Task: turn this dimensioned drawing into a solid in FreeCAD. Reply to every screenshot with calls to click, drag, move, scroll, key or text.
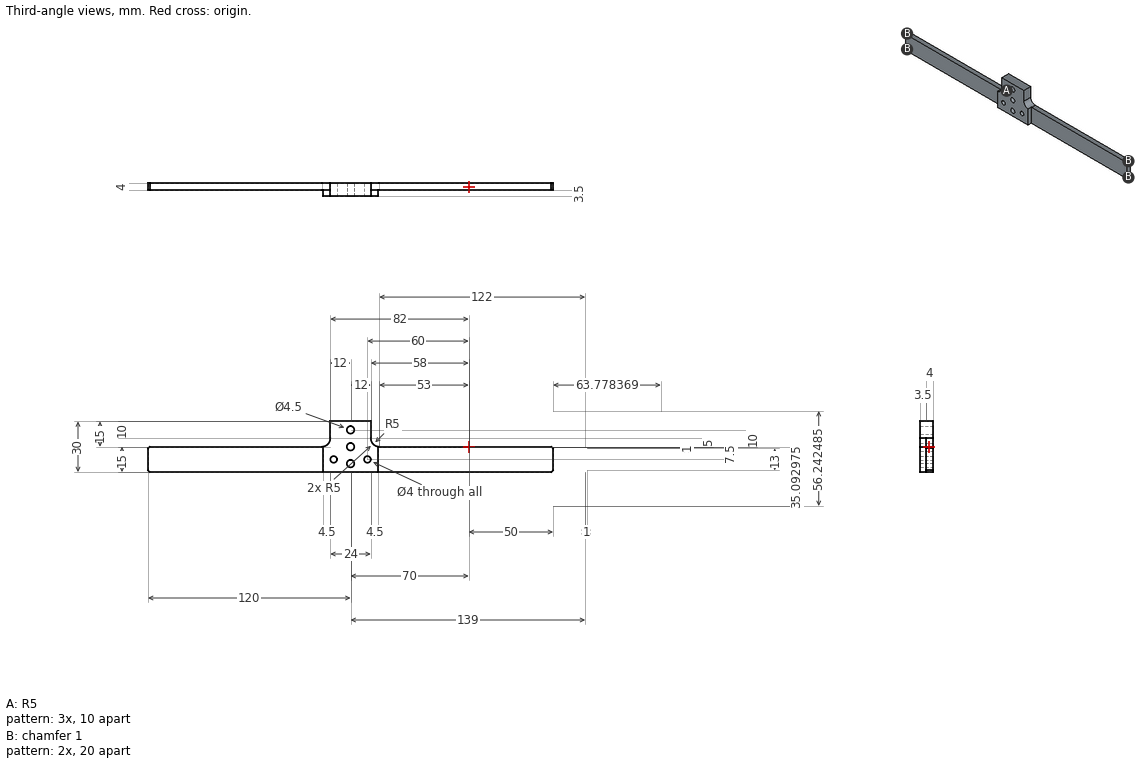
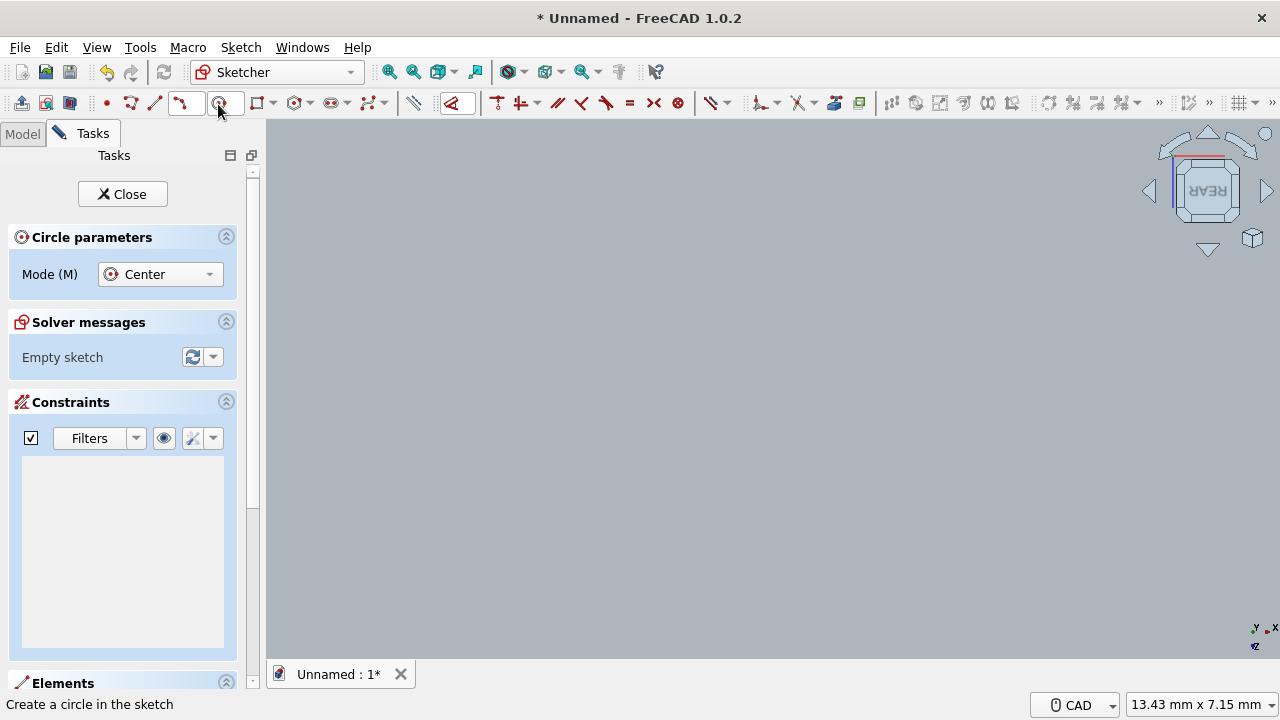
click(704, 389)
click(824, 269)
key(Escape)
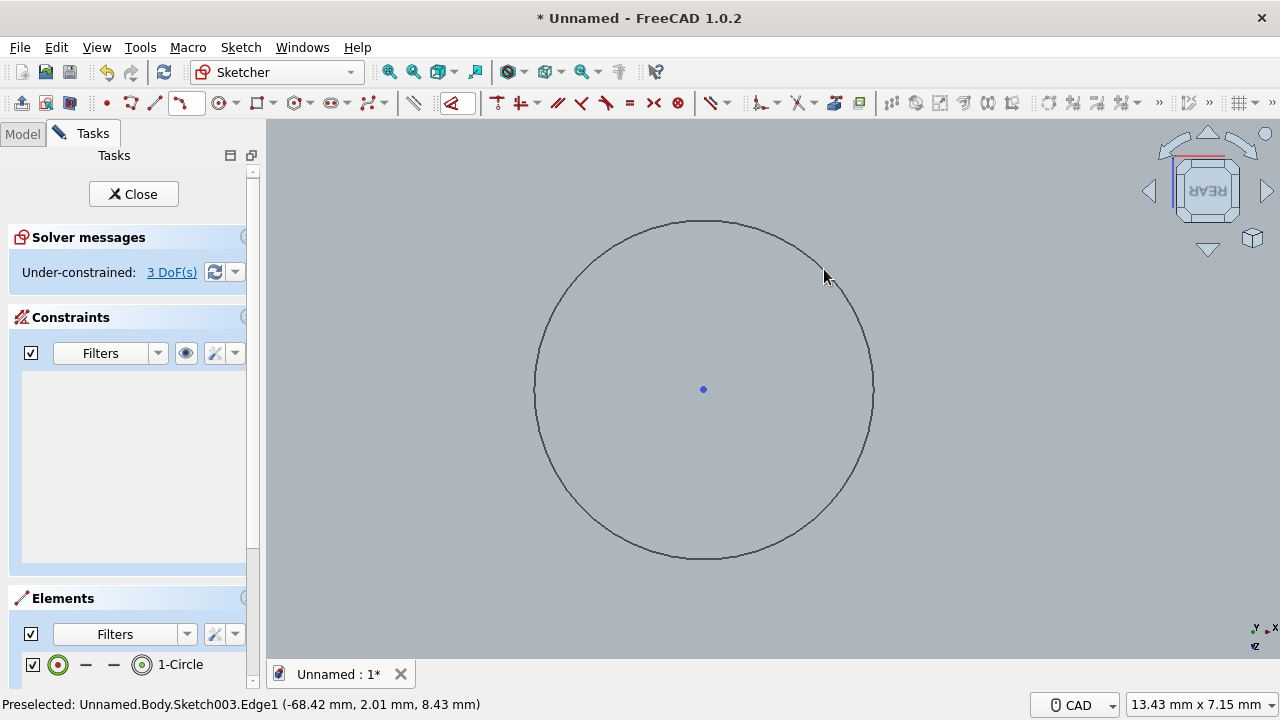
click(824, 270)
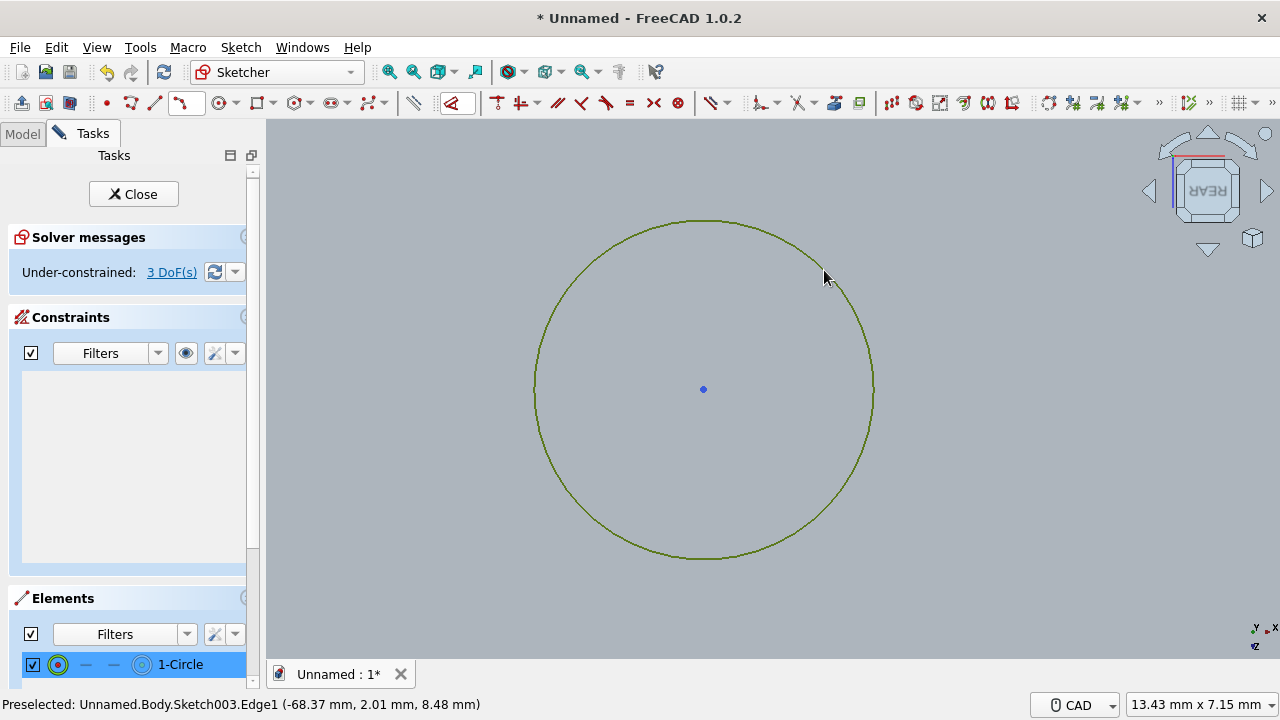
key(k)
key(o)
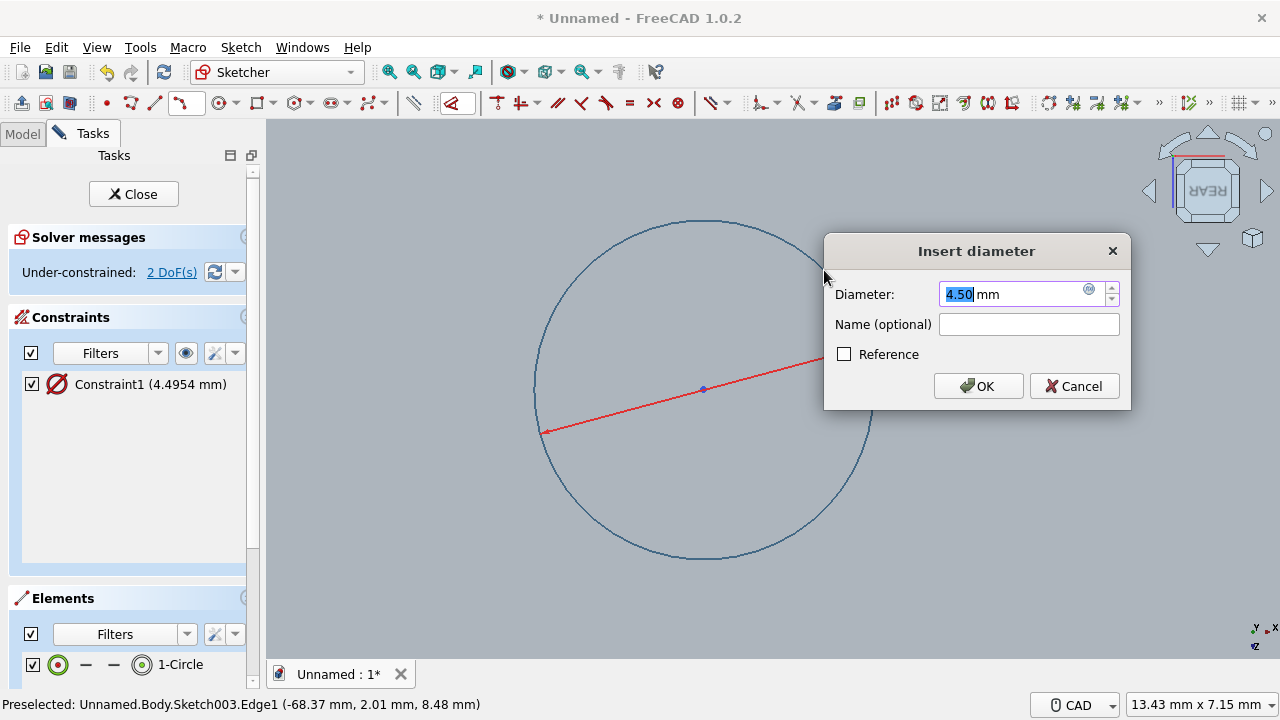
text(4.5)
key(Return)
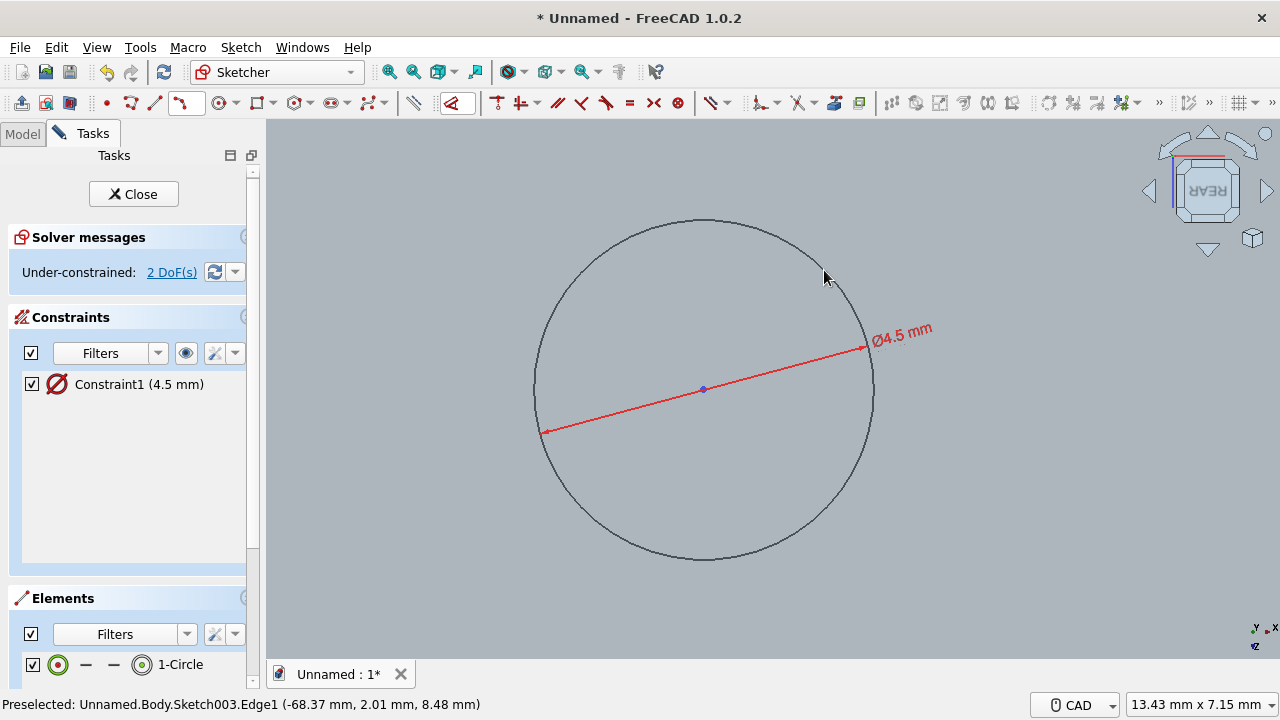
click(704, 390)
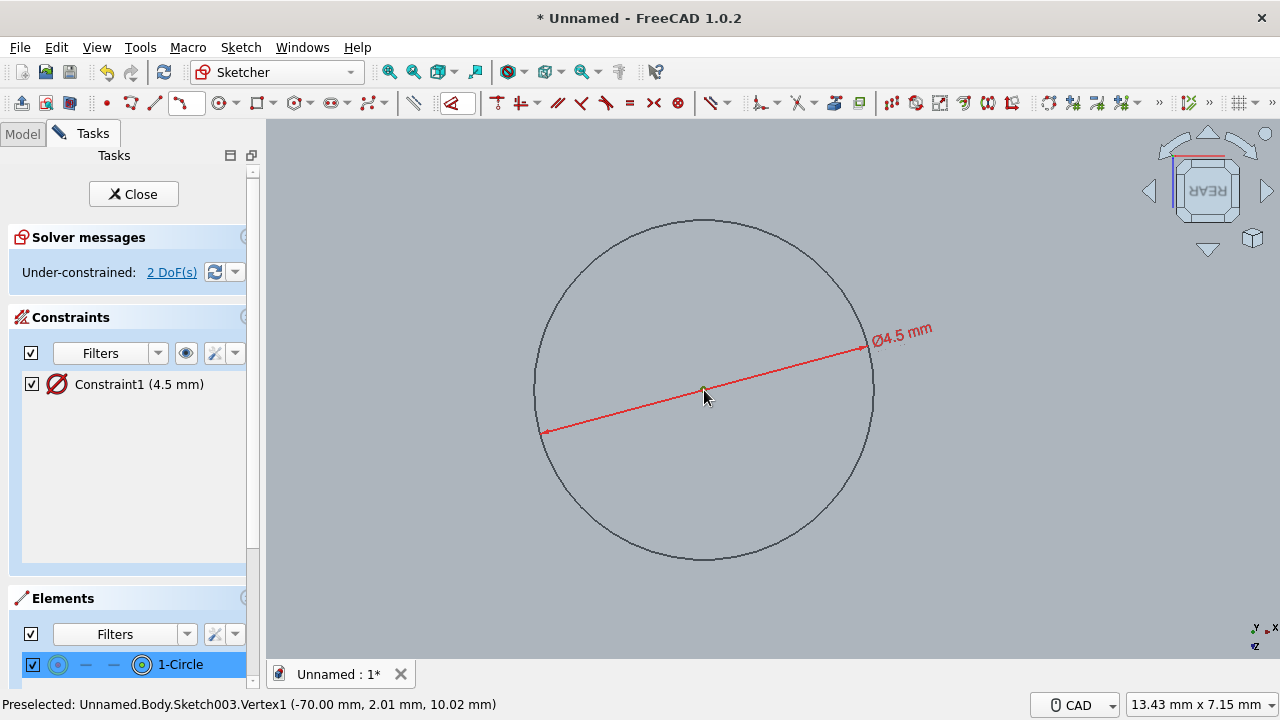
click(470, 104)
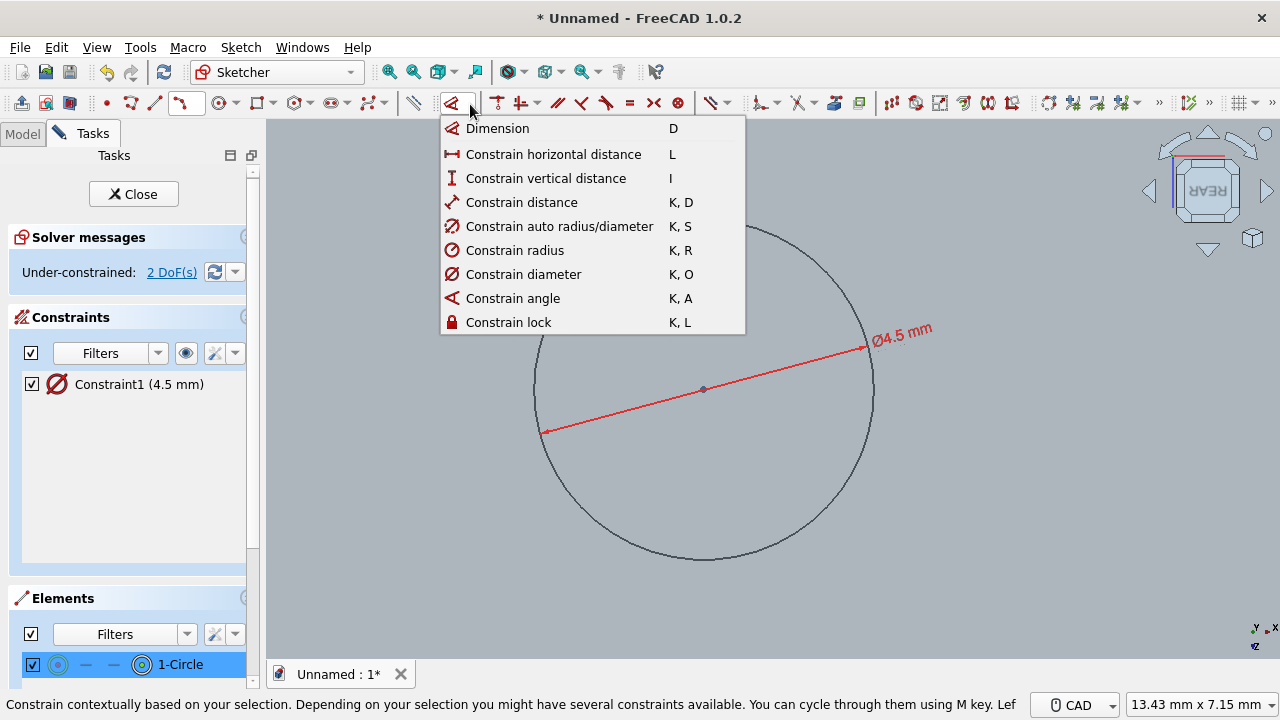
click(593, 154)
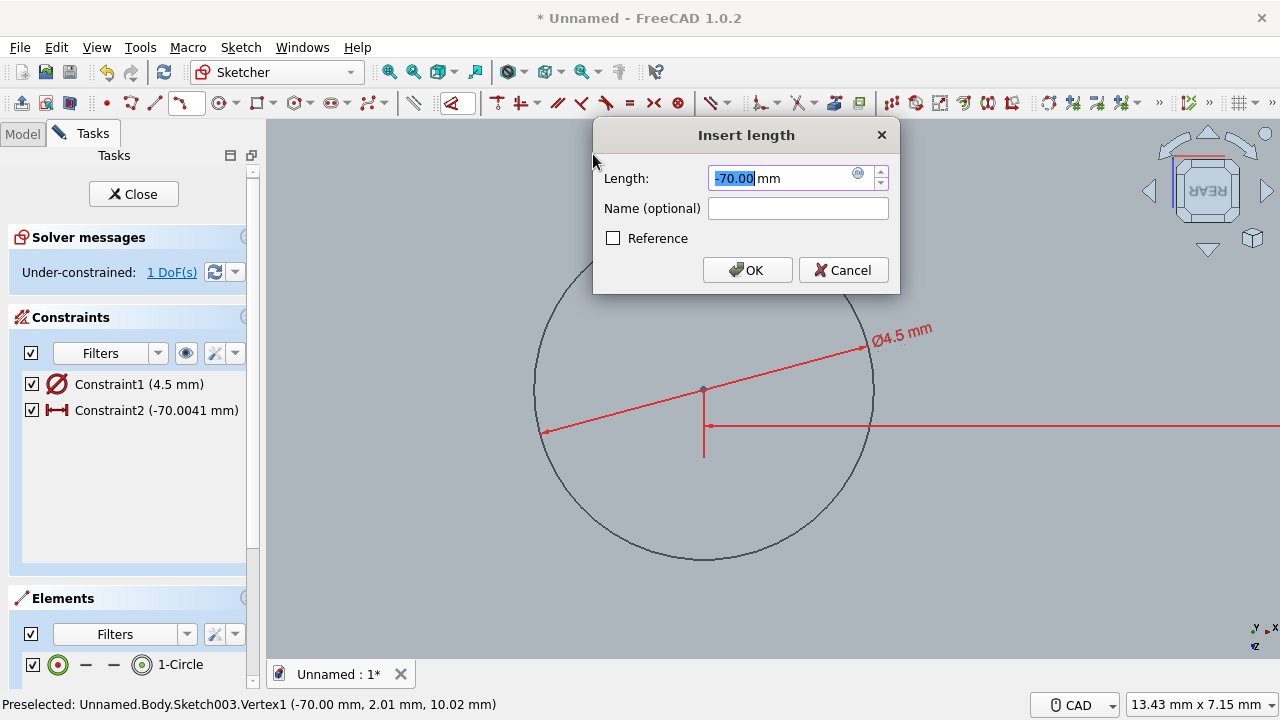
text(-70)
key(Return)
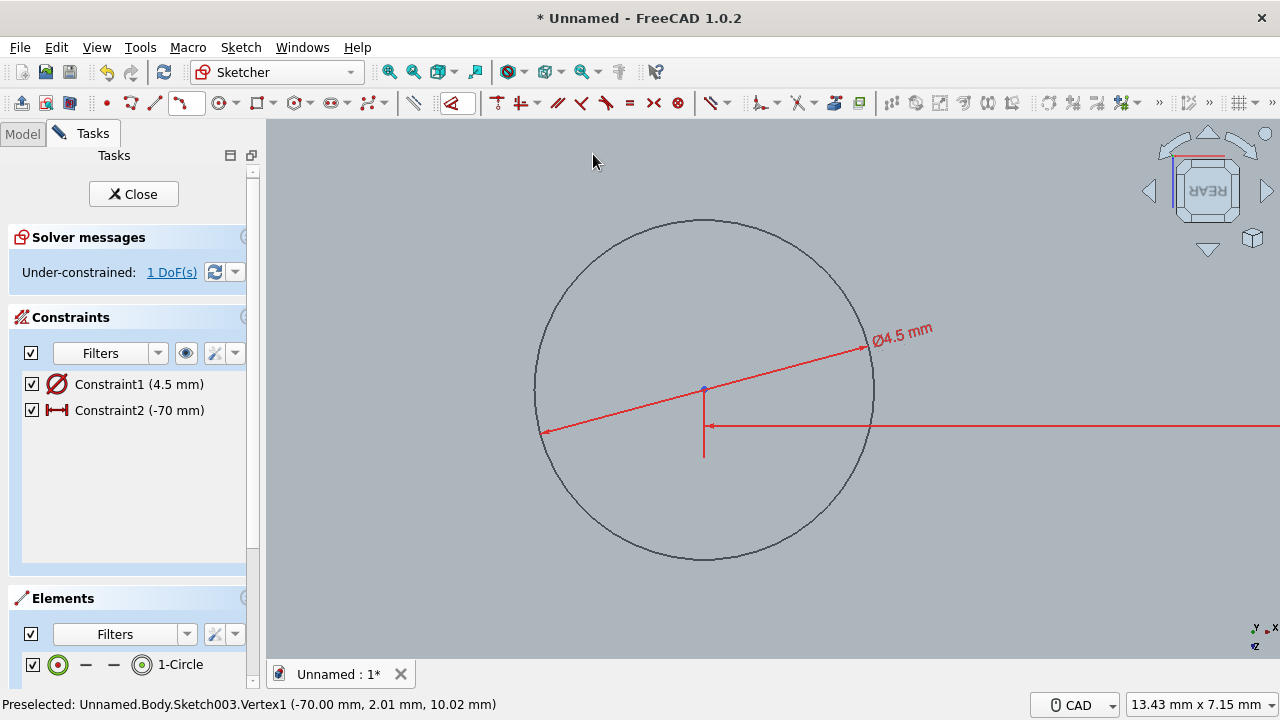
click(704, 390)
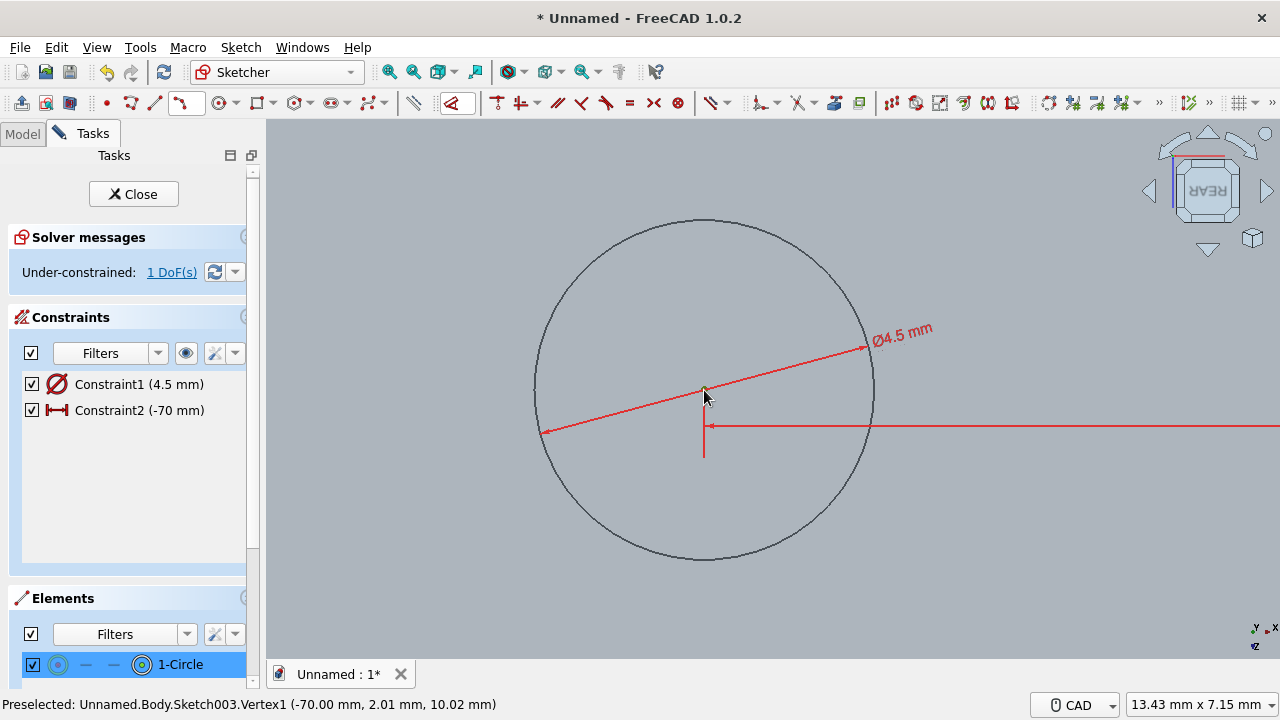
key(i)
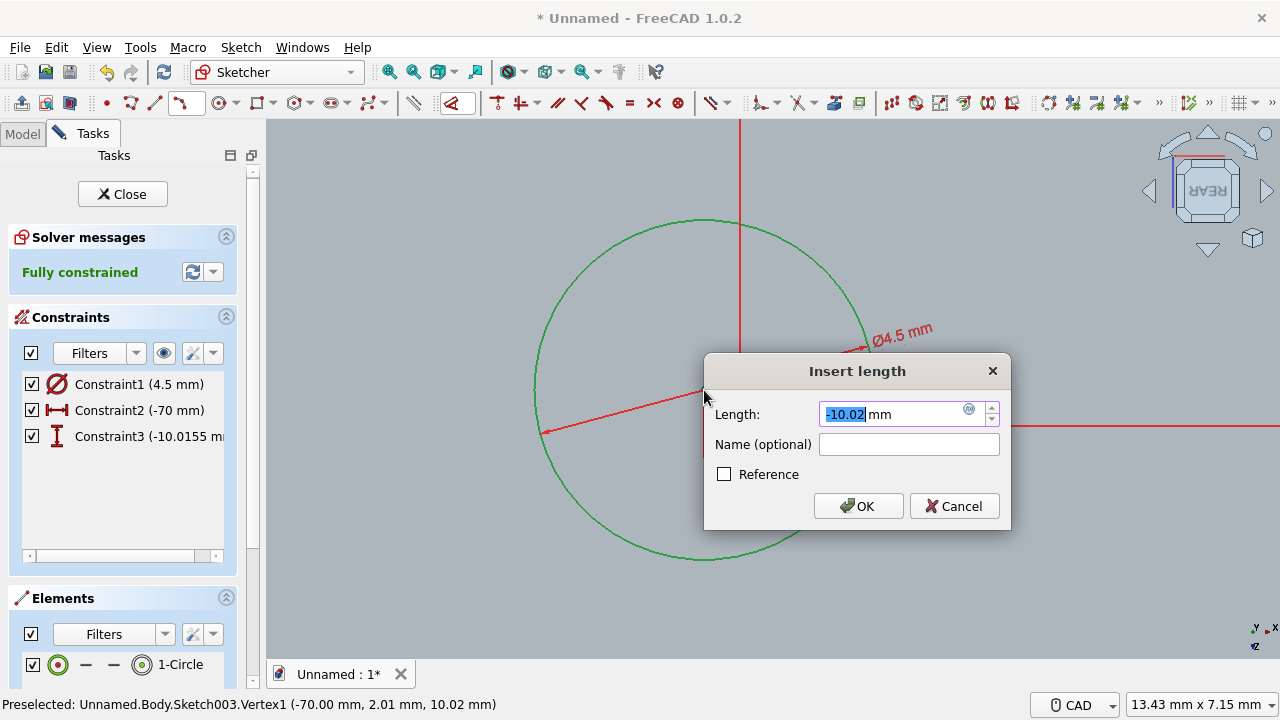
text(-10)
key(Return)